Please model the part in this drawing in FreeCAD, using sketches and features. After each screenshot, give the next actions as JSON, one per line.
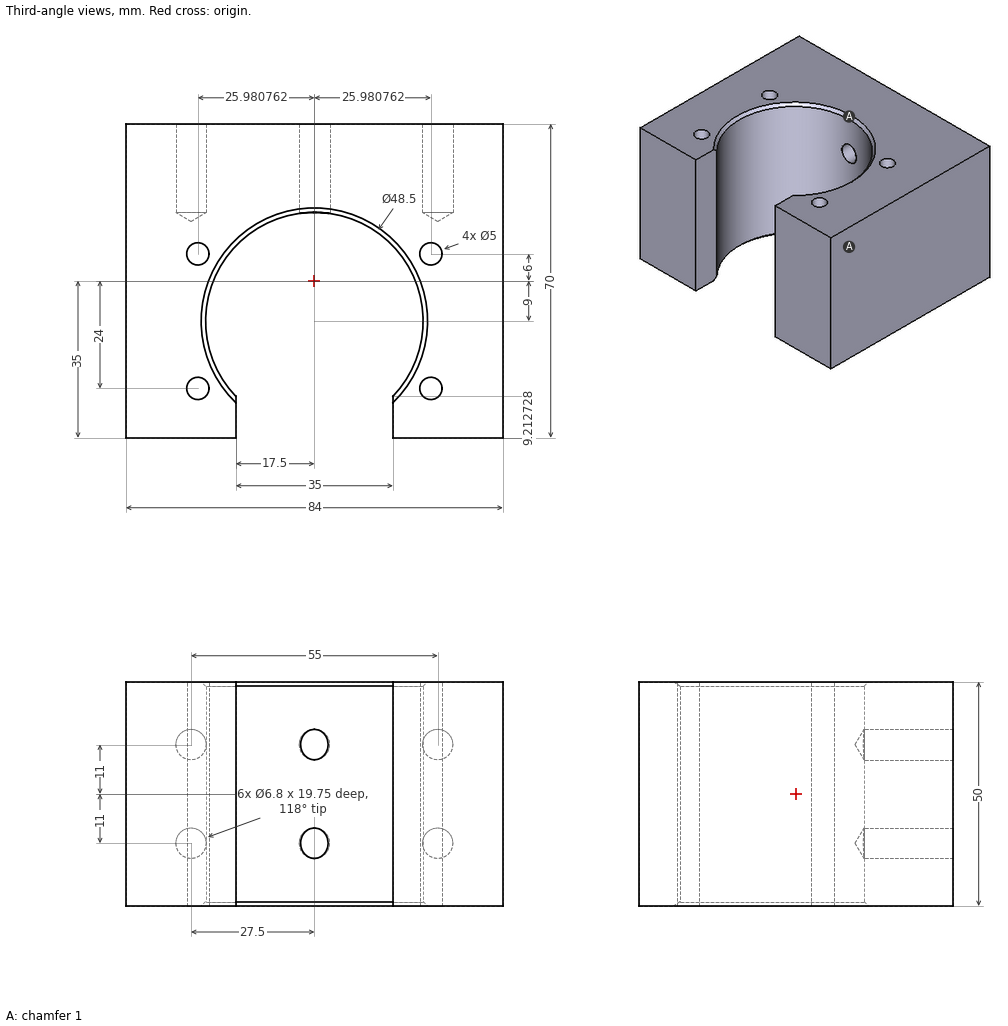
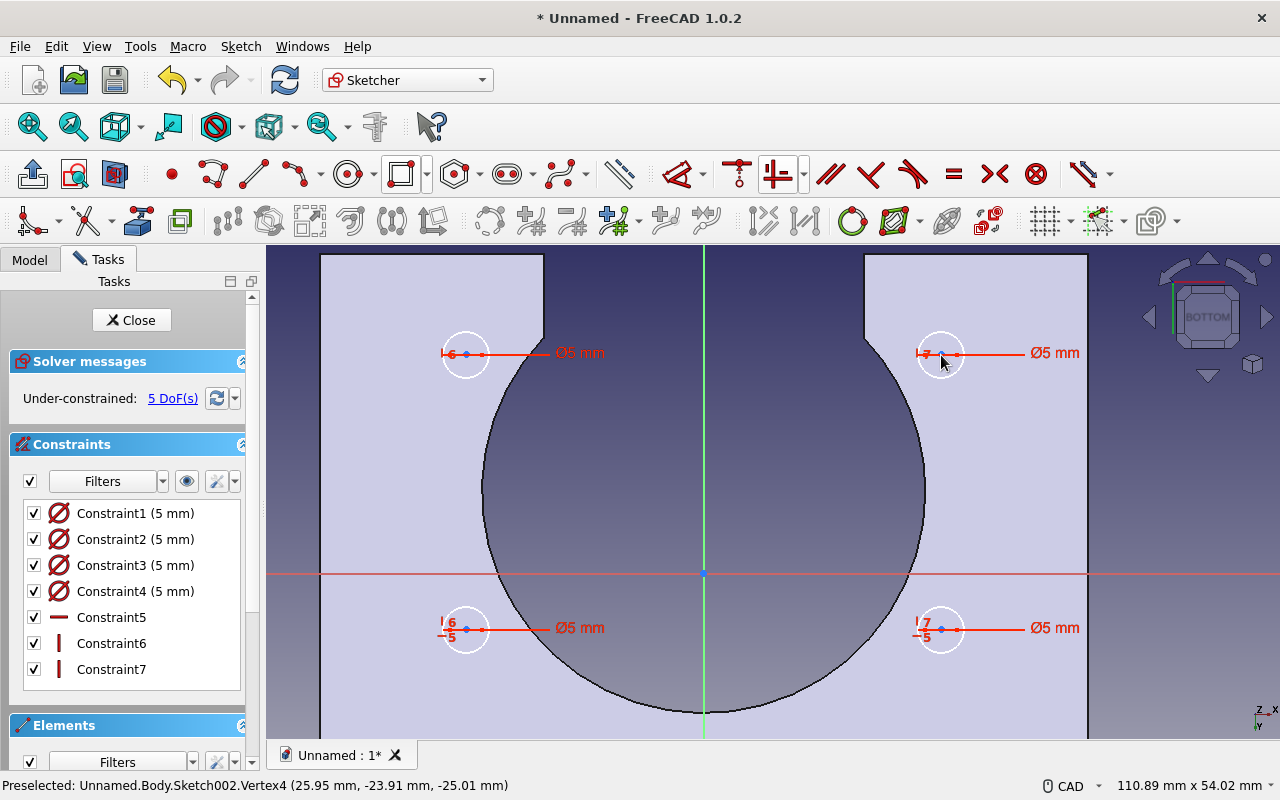
{"action": "left_click", "coordinate": [466, 355]}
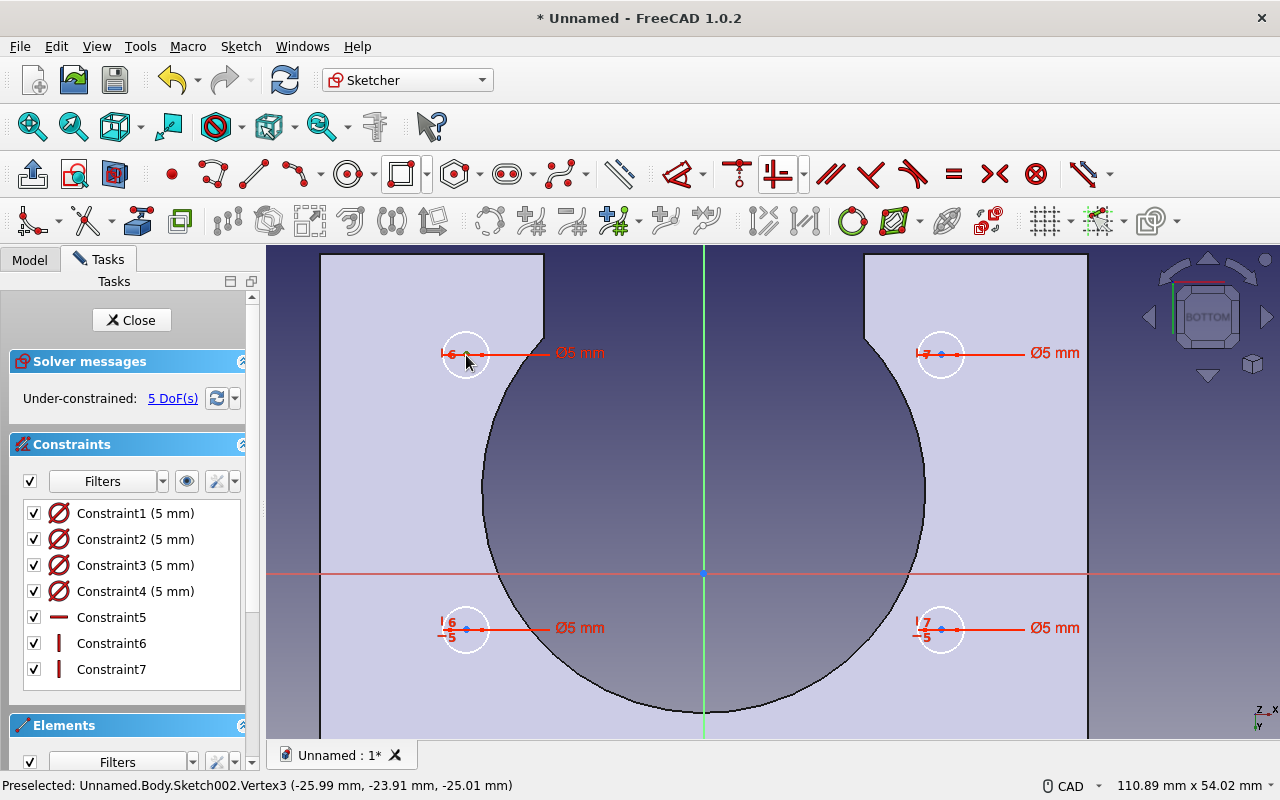
{"action": "left_click", "coordinate": [941, 355]}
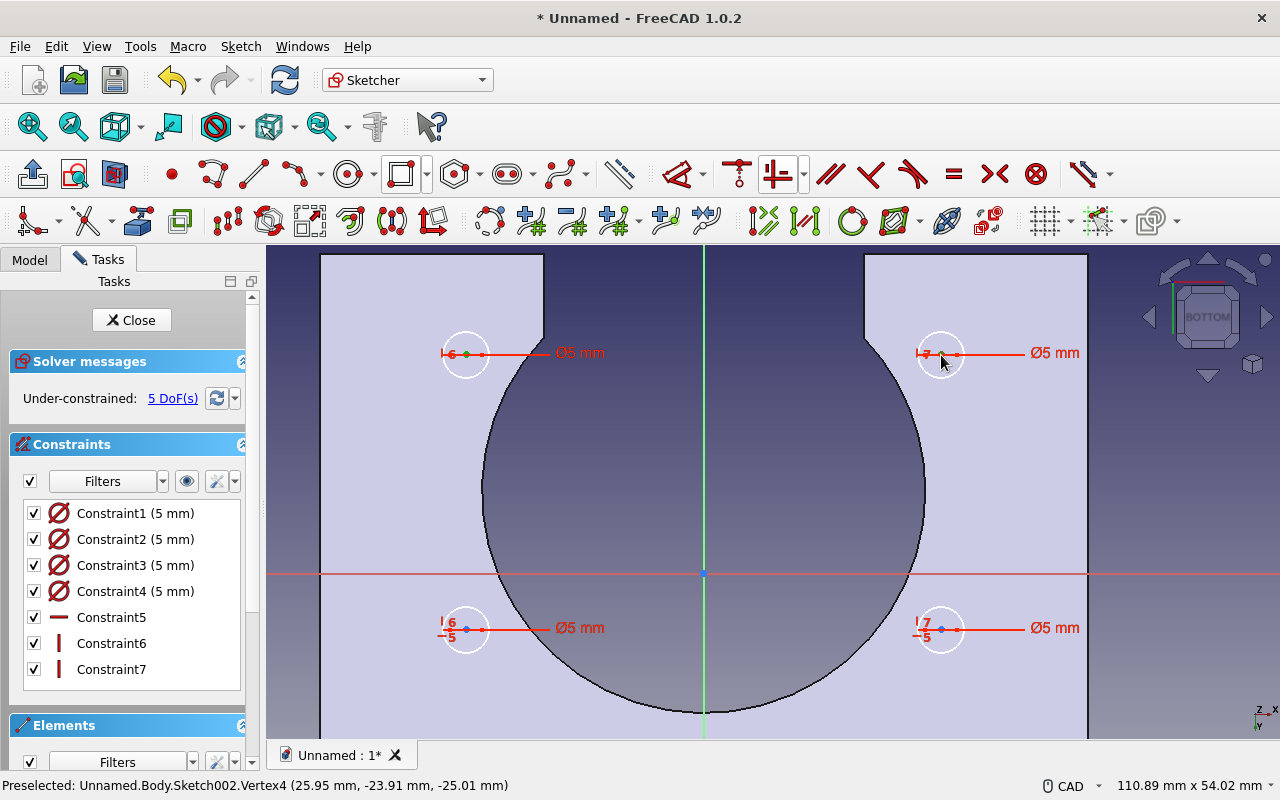
{"action": "key", "text": "h"}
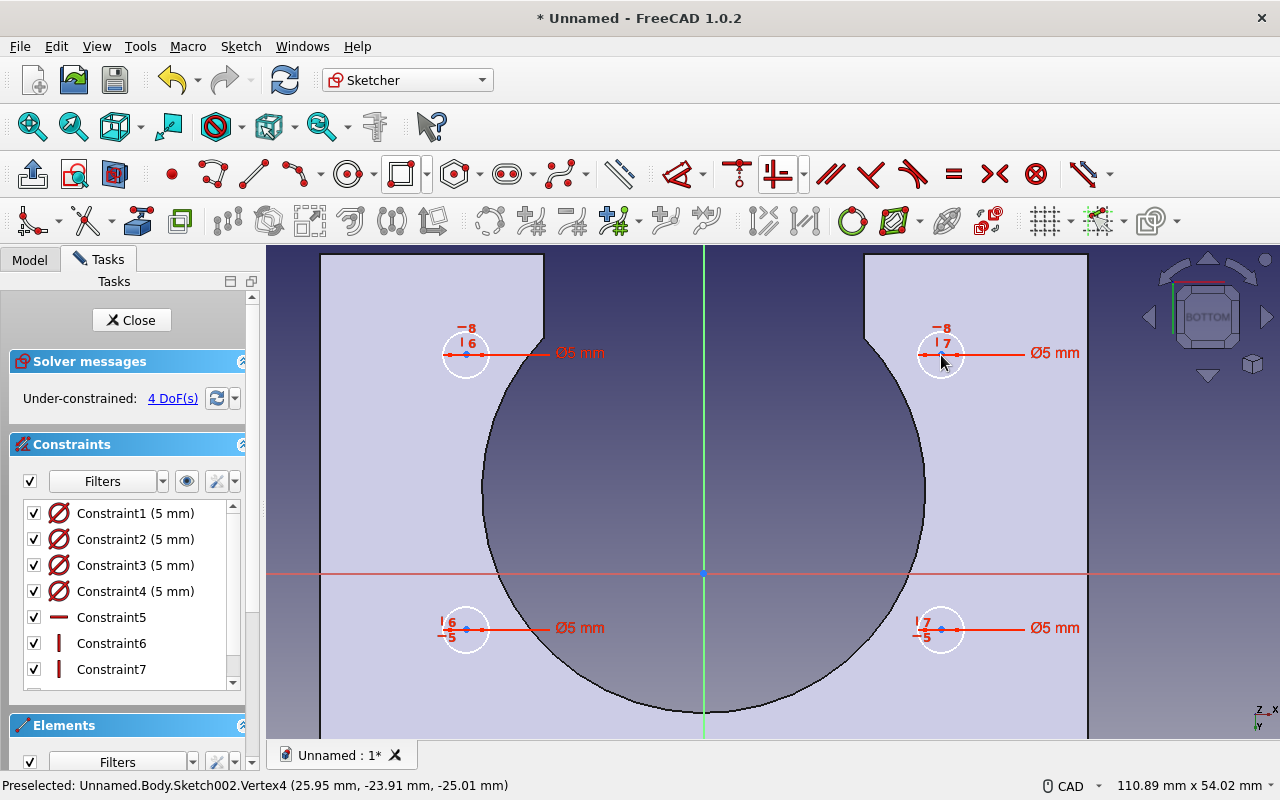
{"action": "left_click", "coordinate": [676, 174]}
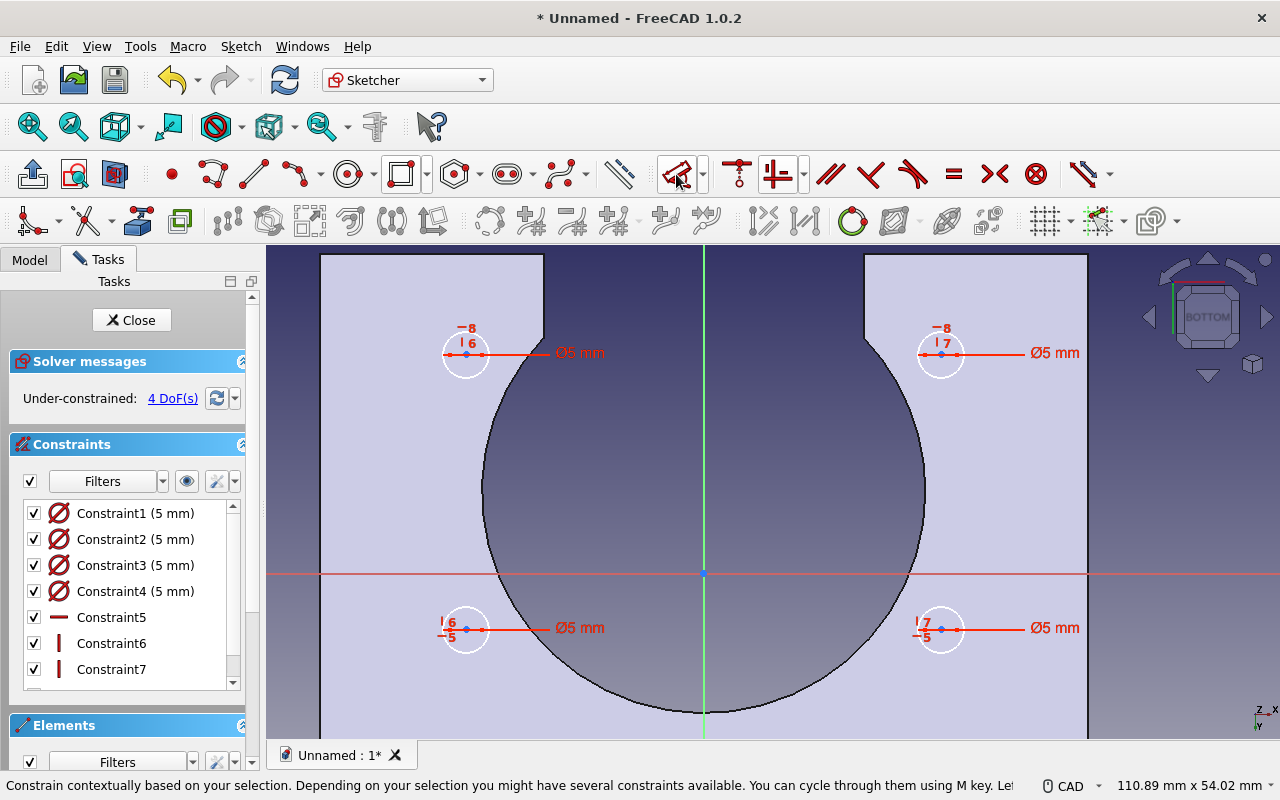
{"action": "left_click", "coordinate": [941, 630]}
{"action": "left_click", "coordinate": [975, 602]}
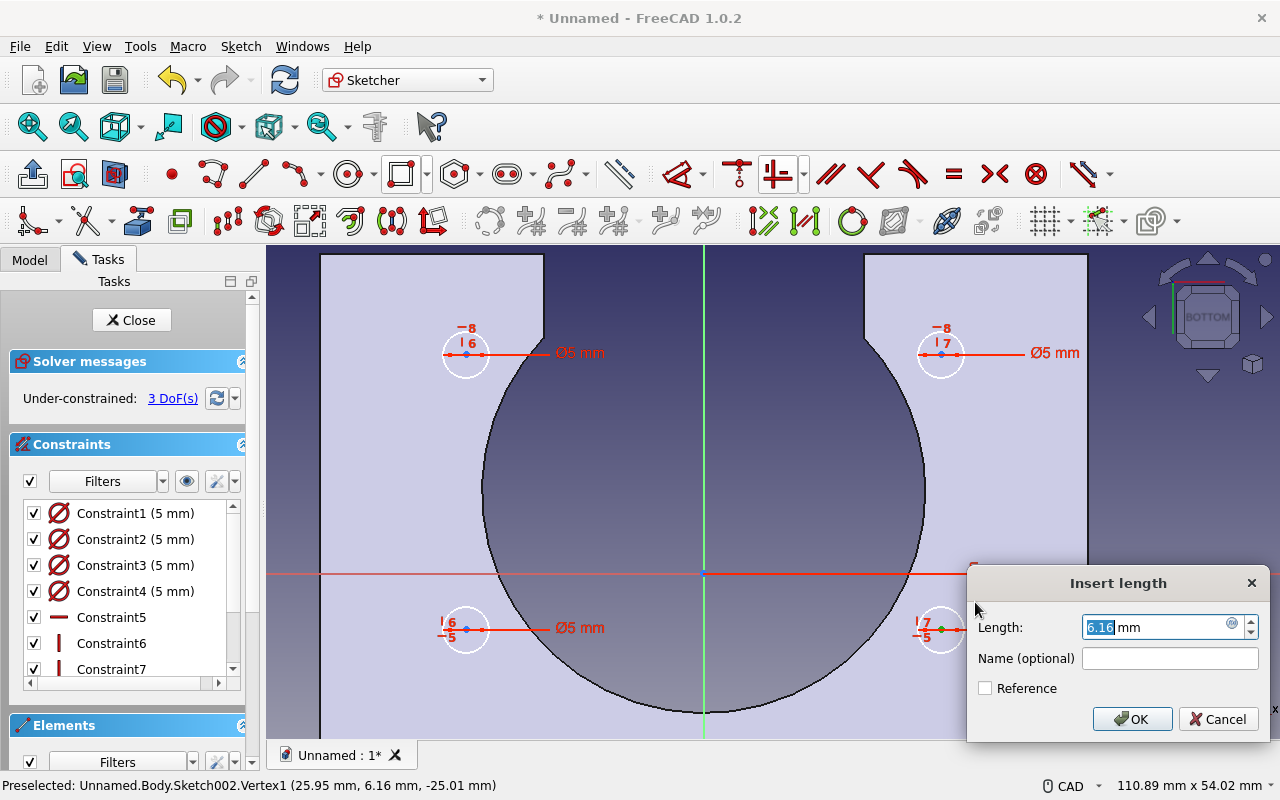
{"action": "type", "text": "6"}
{"action": "key", "text": "Return"}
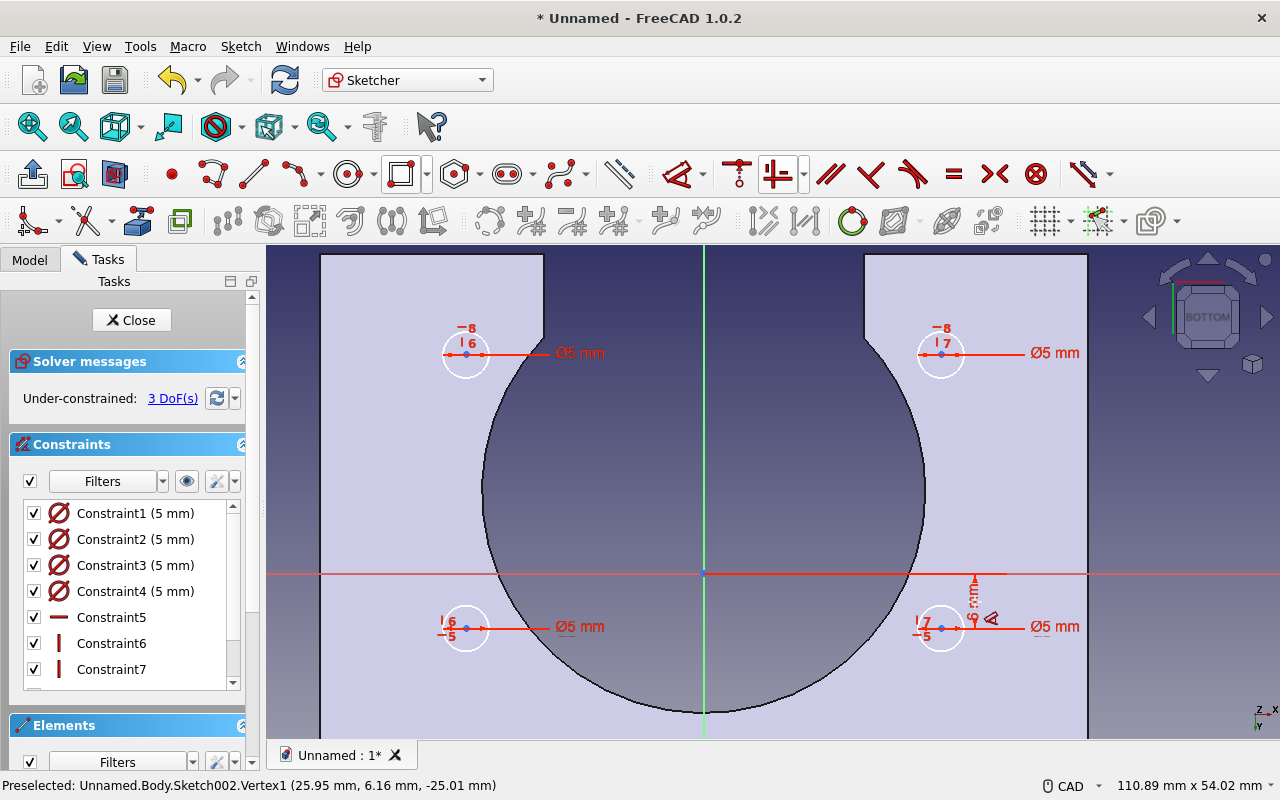
{"action": "left_click", "coordinate": [466, 355]}
{"action": "left_click", "coordinate": [432, 464]}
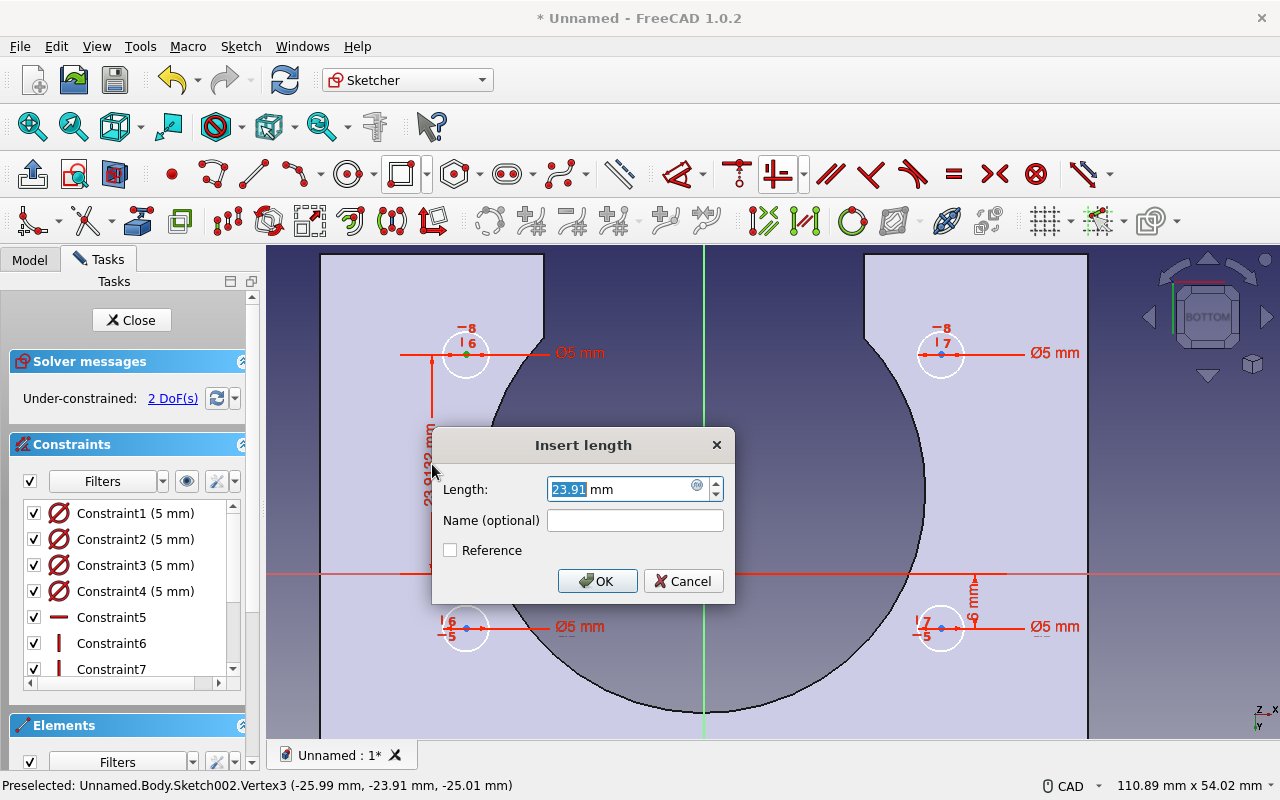
{"action": "type", "text": "24"}
{"action": "key", "text": "Return"}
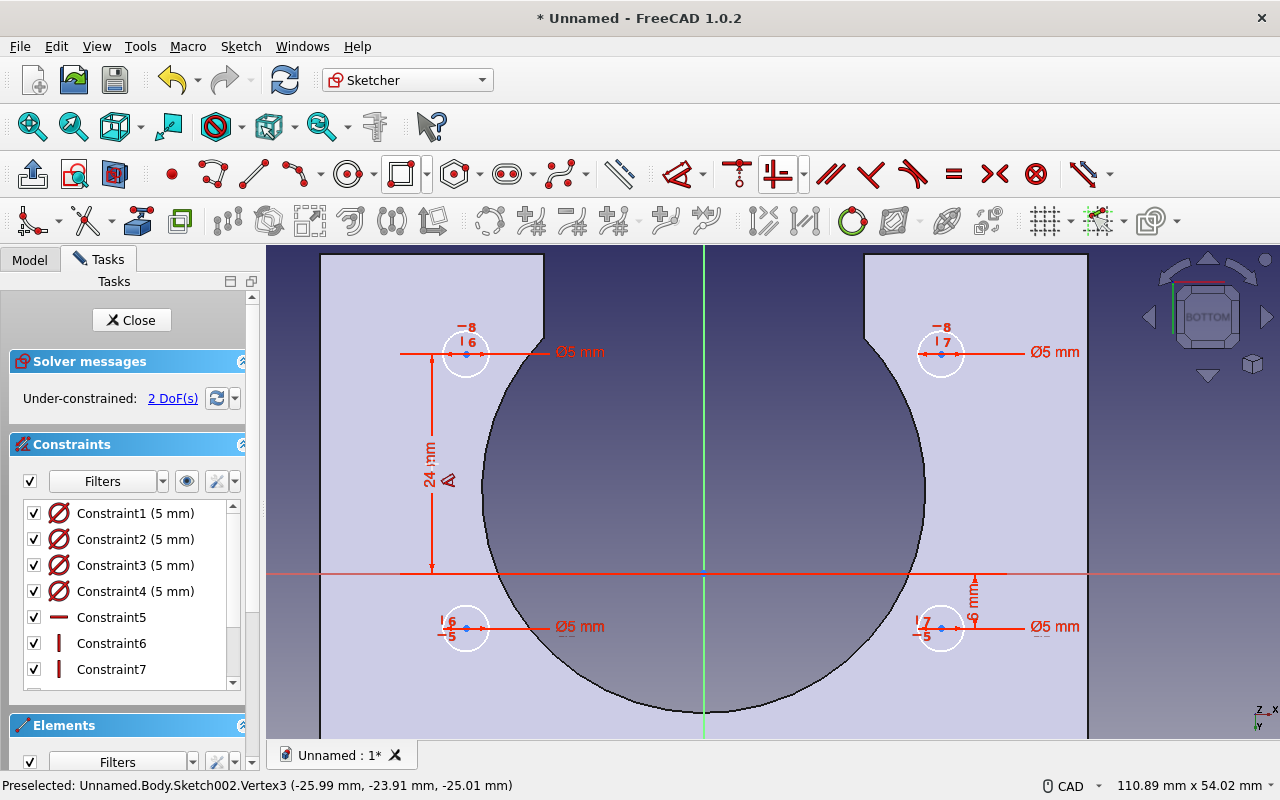
{"action": "left_click", "coordinate": [941, 629]}
{"action": "left_click", "coordinate": [822, 663]}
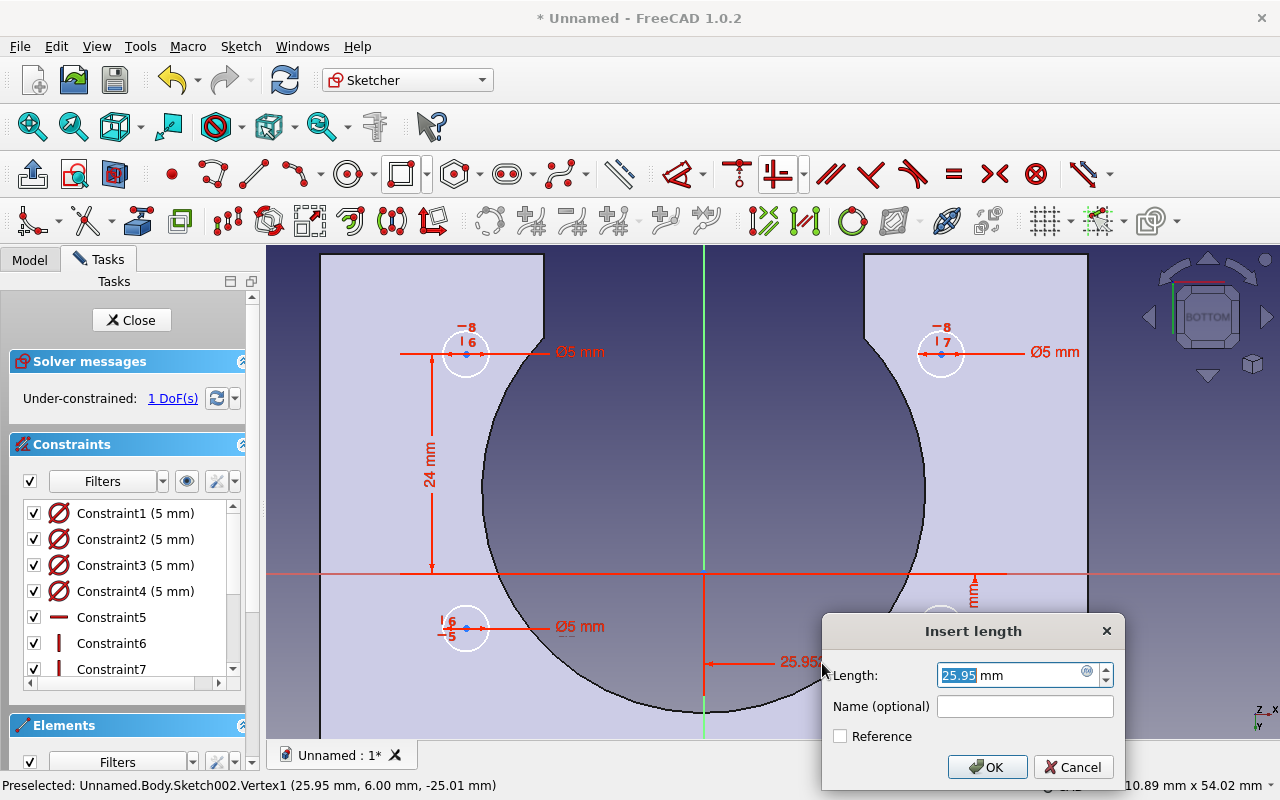
{"action": "type", "text": "25.980762"}
{"action": "key", "text": "Return"}